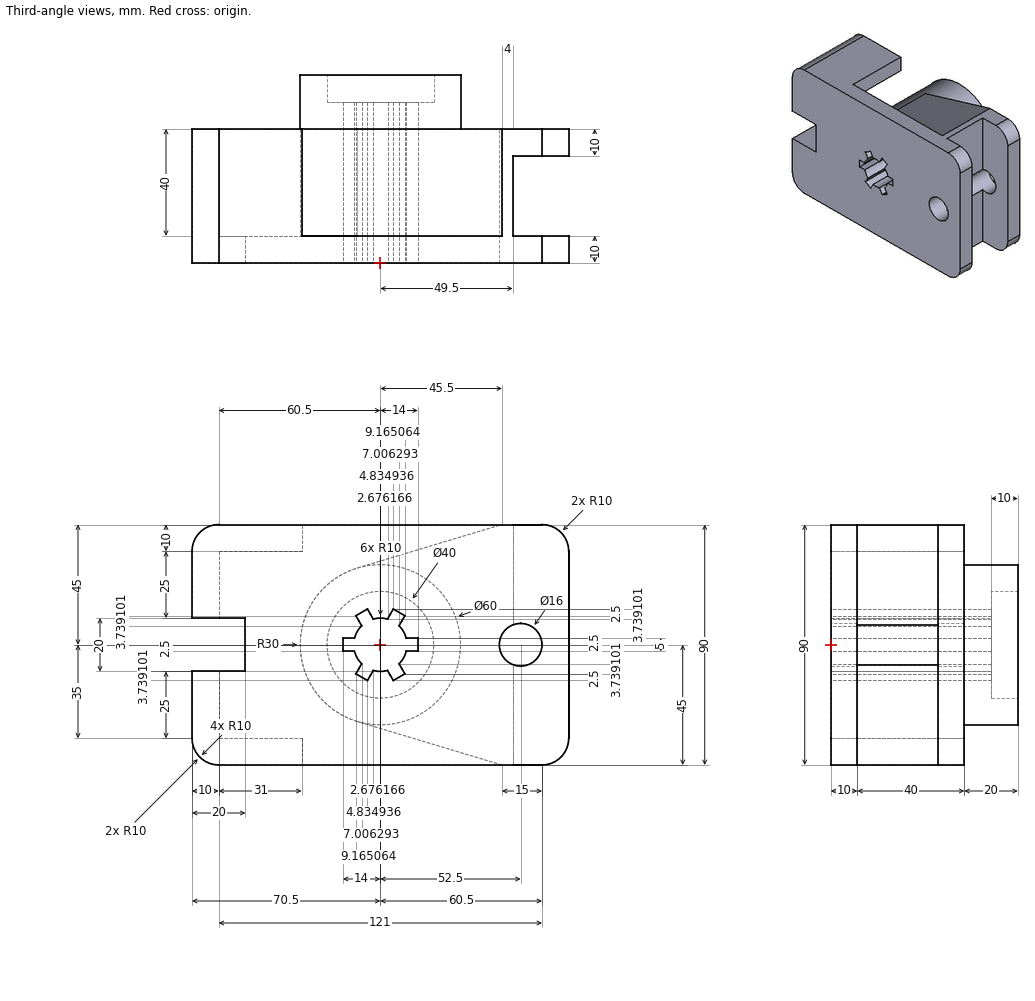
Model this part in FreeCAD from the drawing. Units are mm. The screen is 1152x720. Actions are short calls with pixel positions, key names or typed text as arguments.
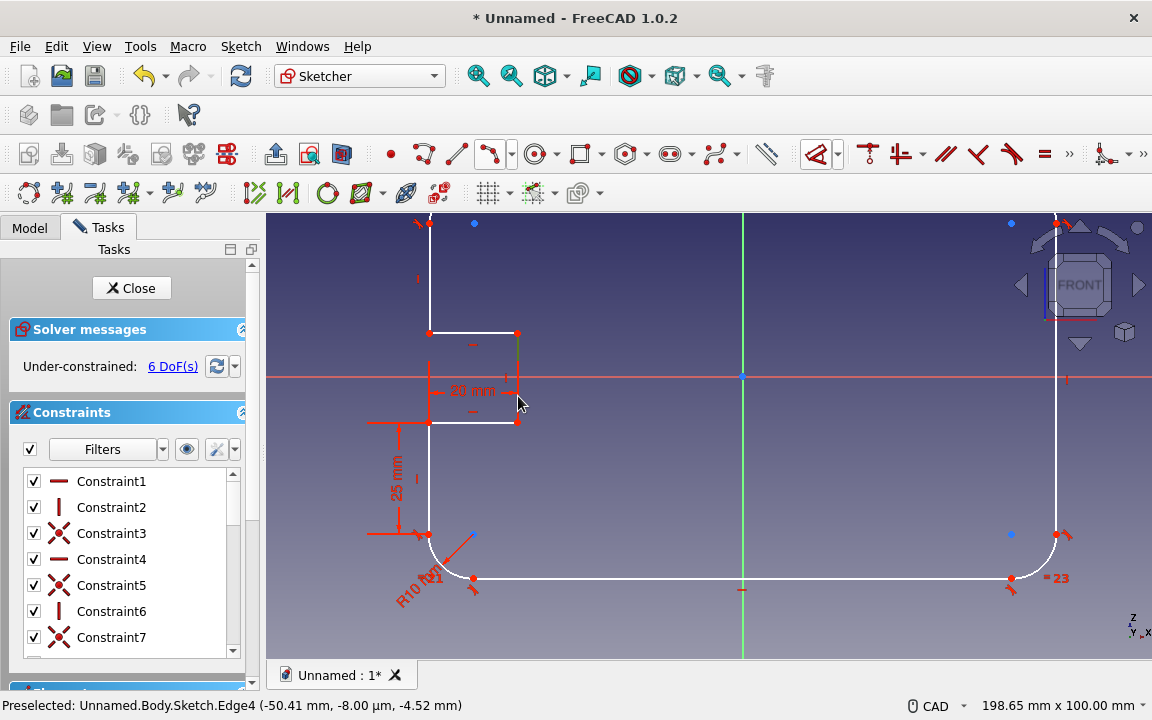
click(838, 154)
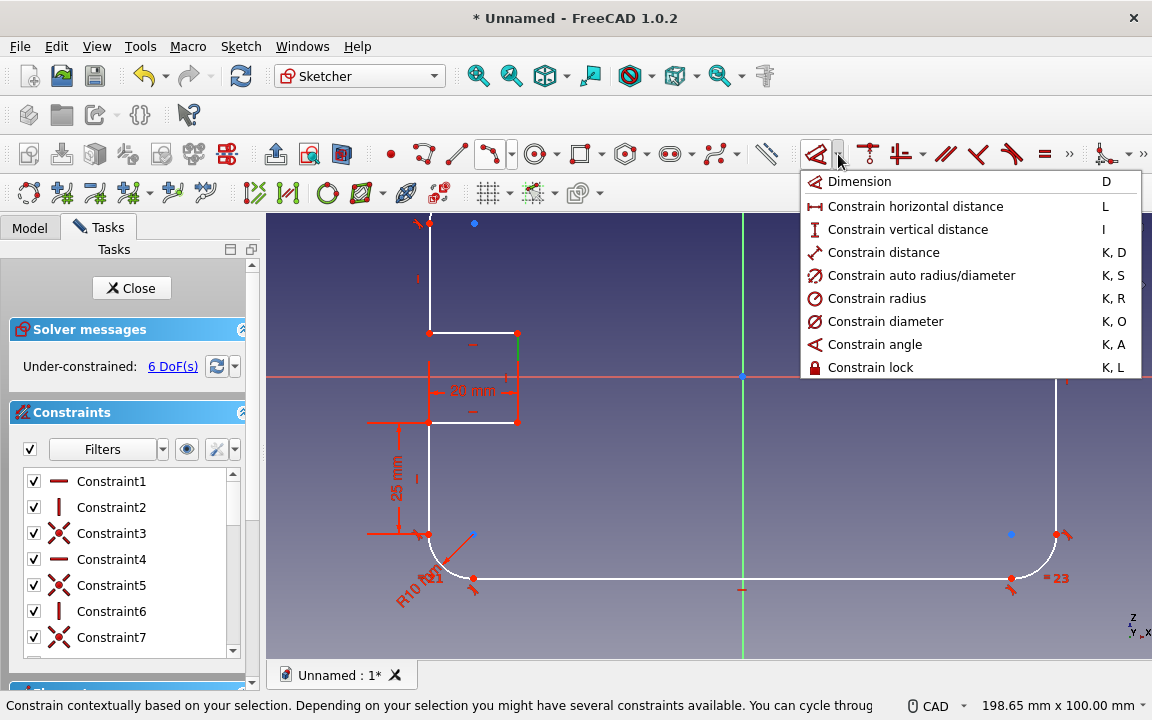
click(971, 230)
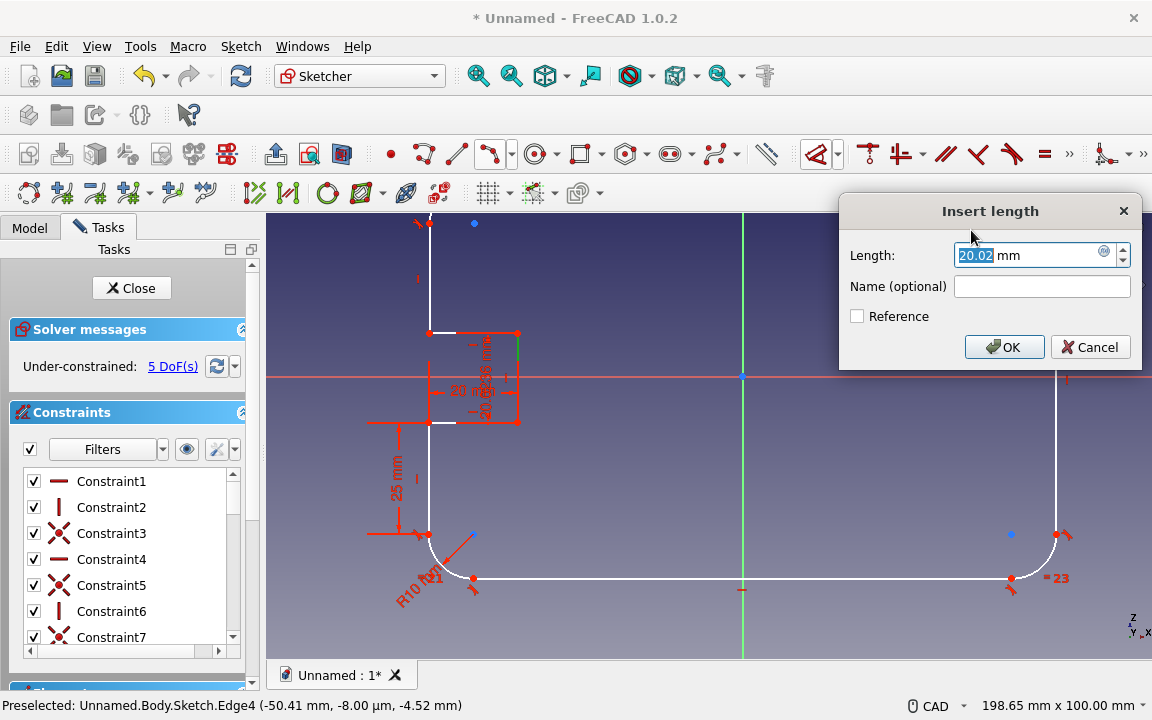
text(20)
key(Return)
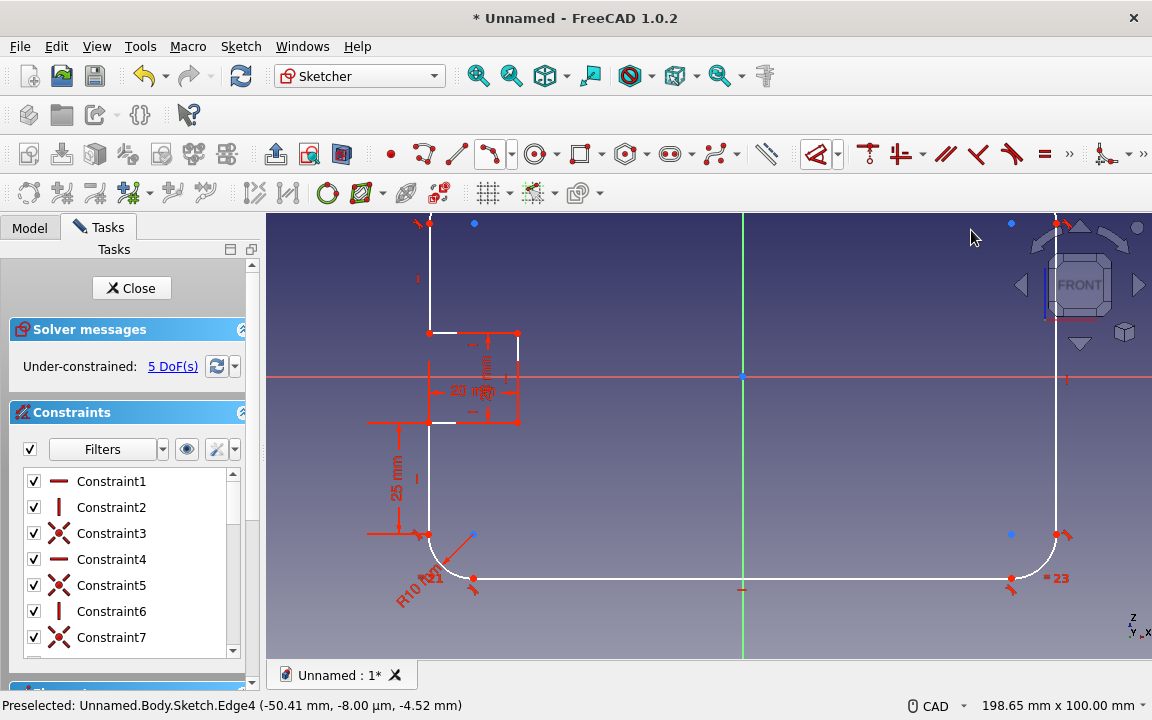
click(491, 333)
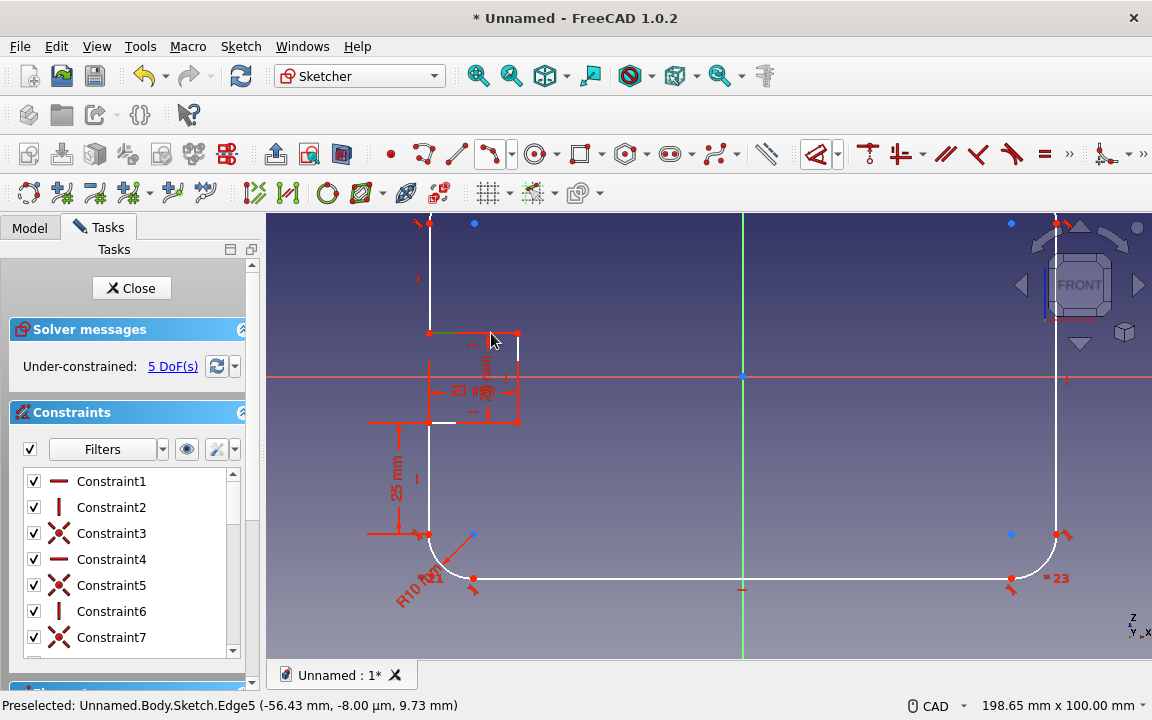
click(838, 154)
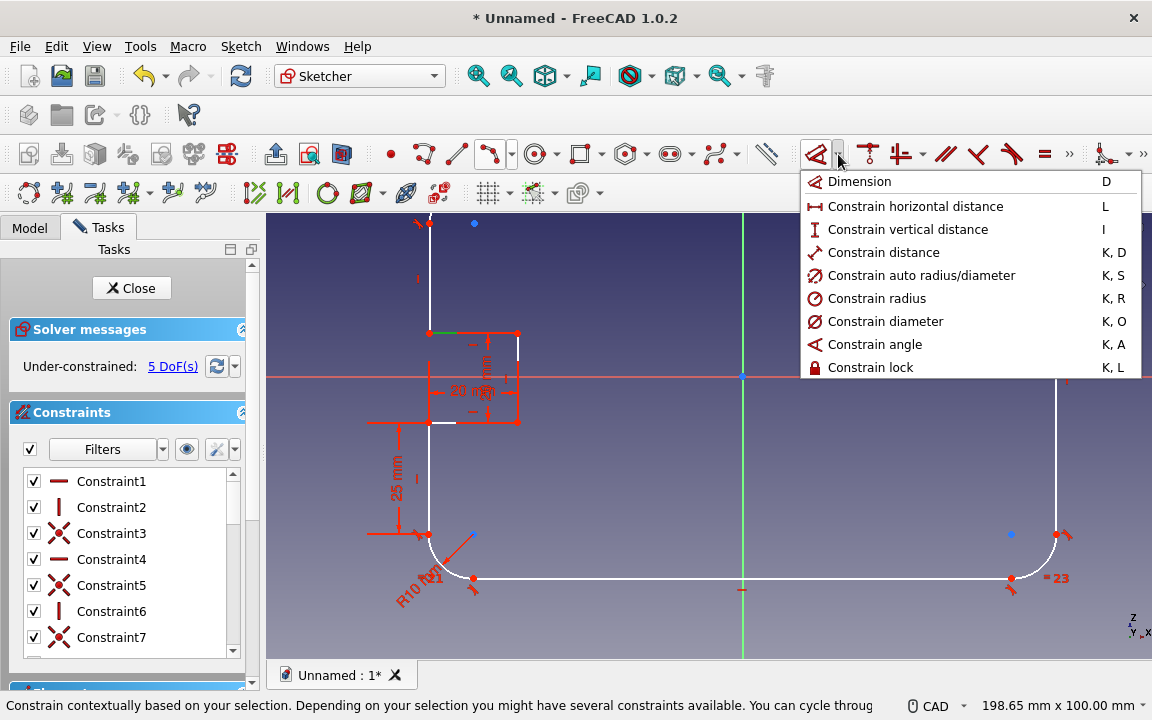
click(971, 206)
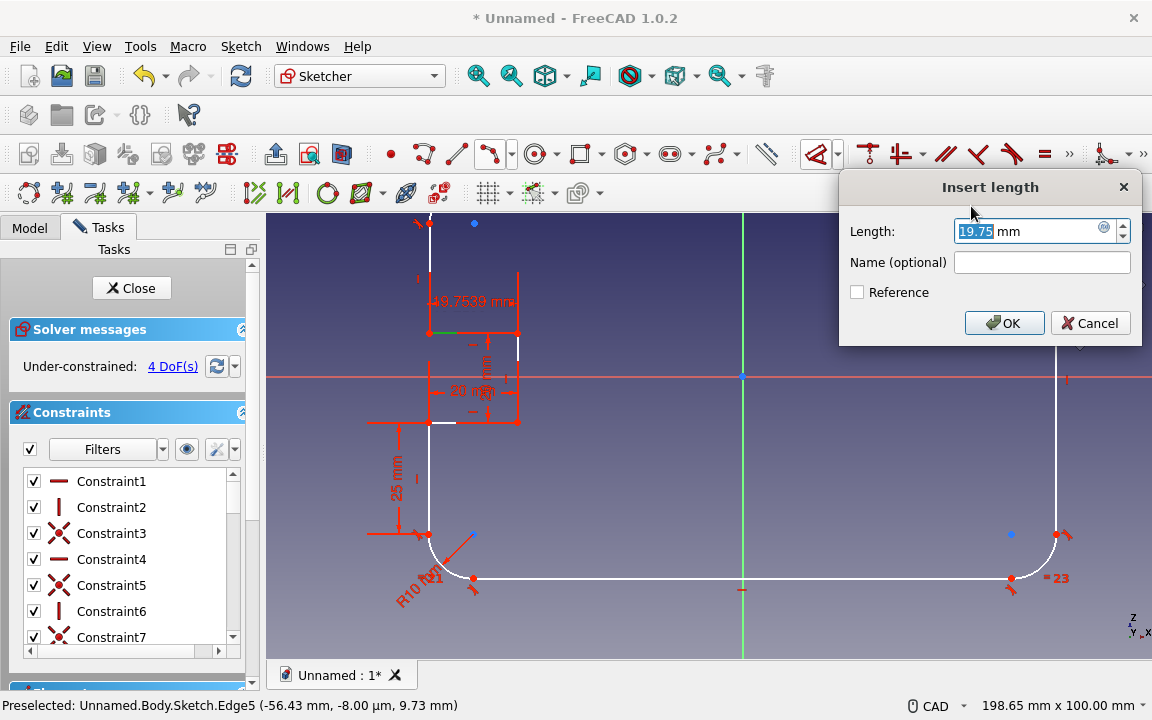
text(20)
key(Return)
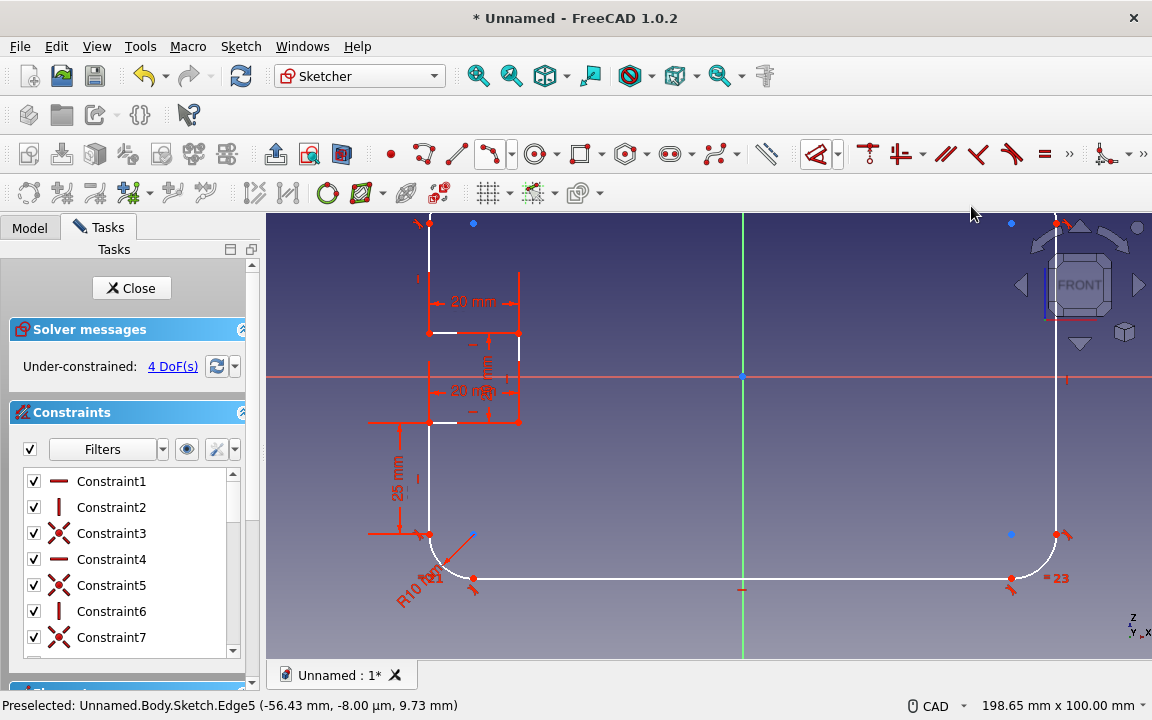
click(429, 301)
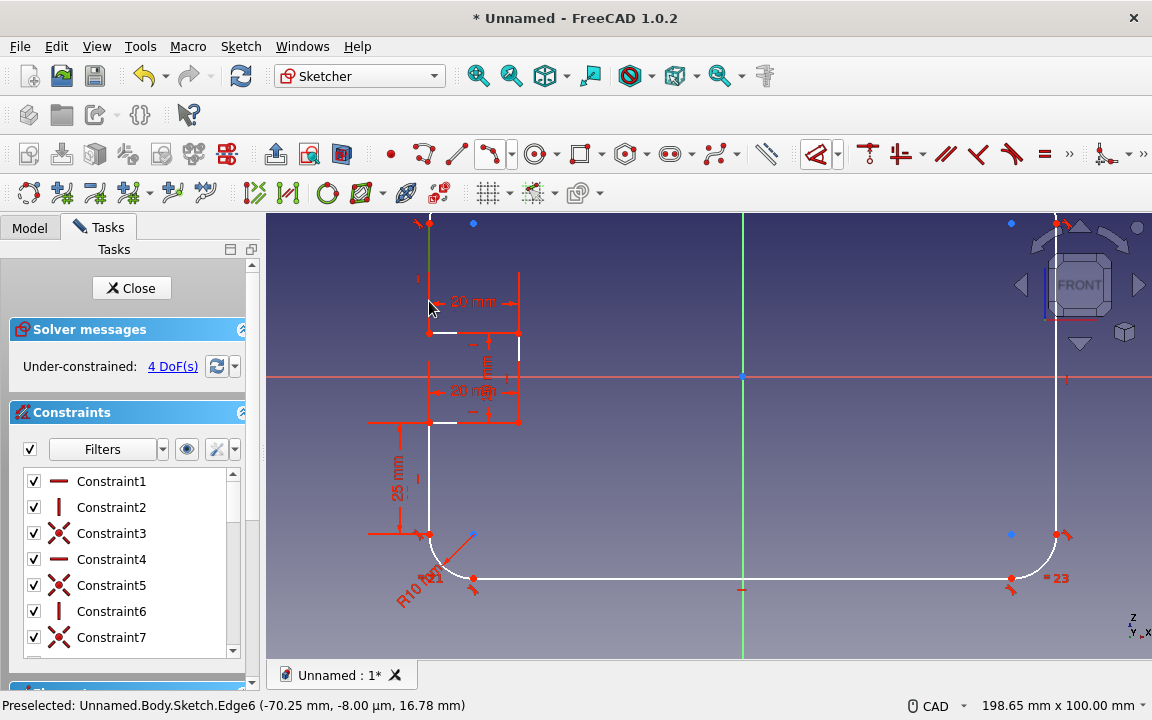
click(838, 154)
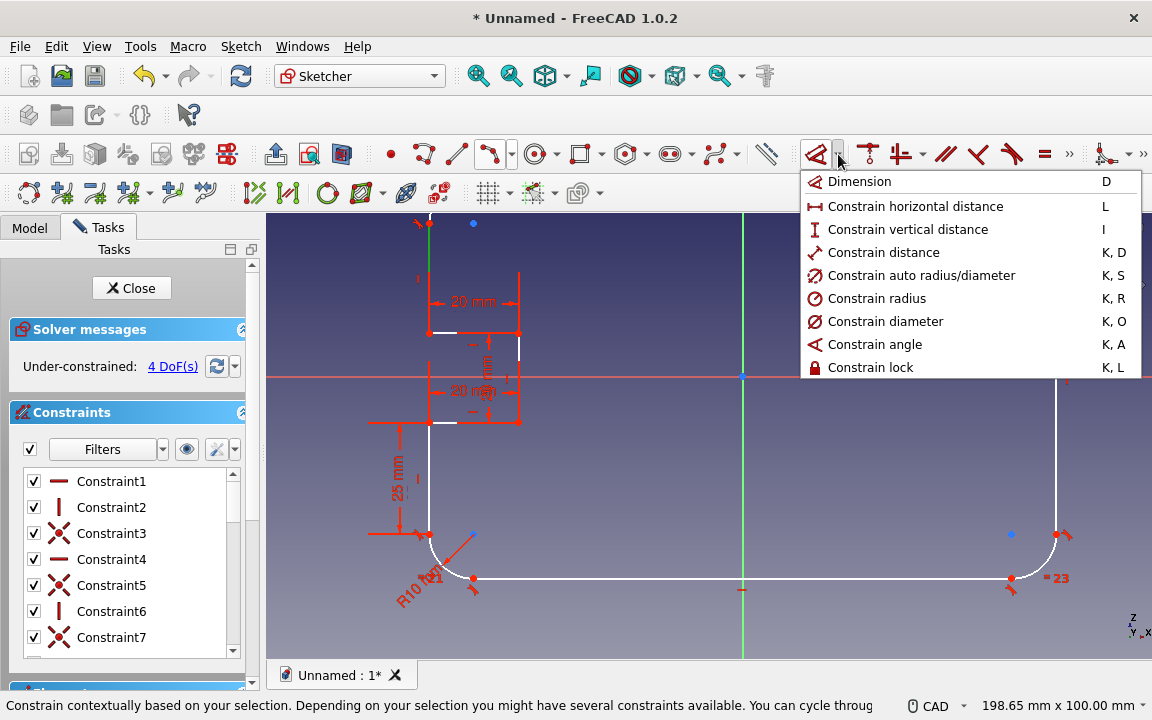
click(971, 230)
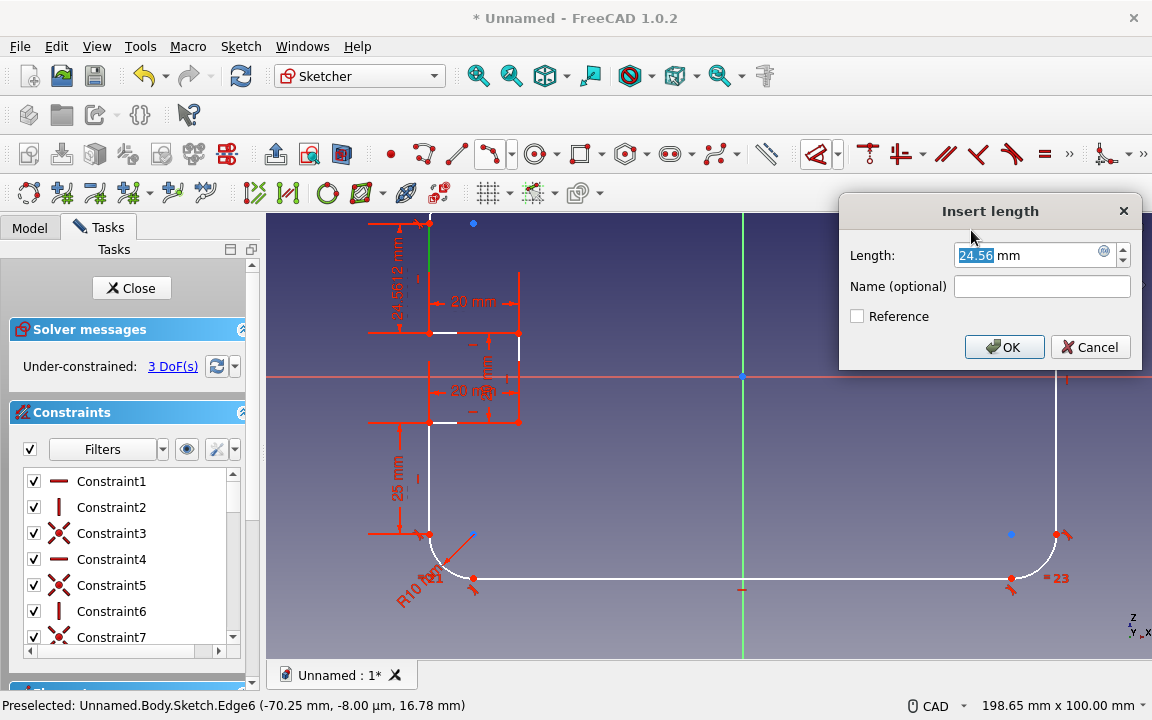
text(25)
key(Return)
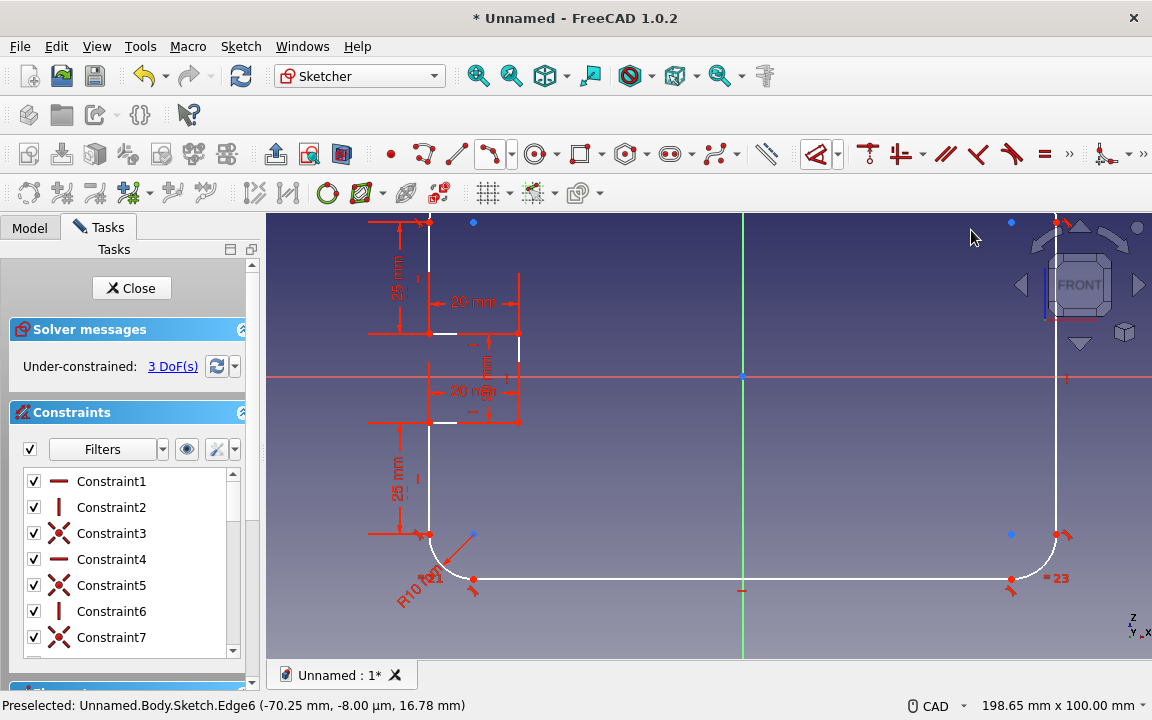
click(850, 579)